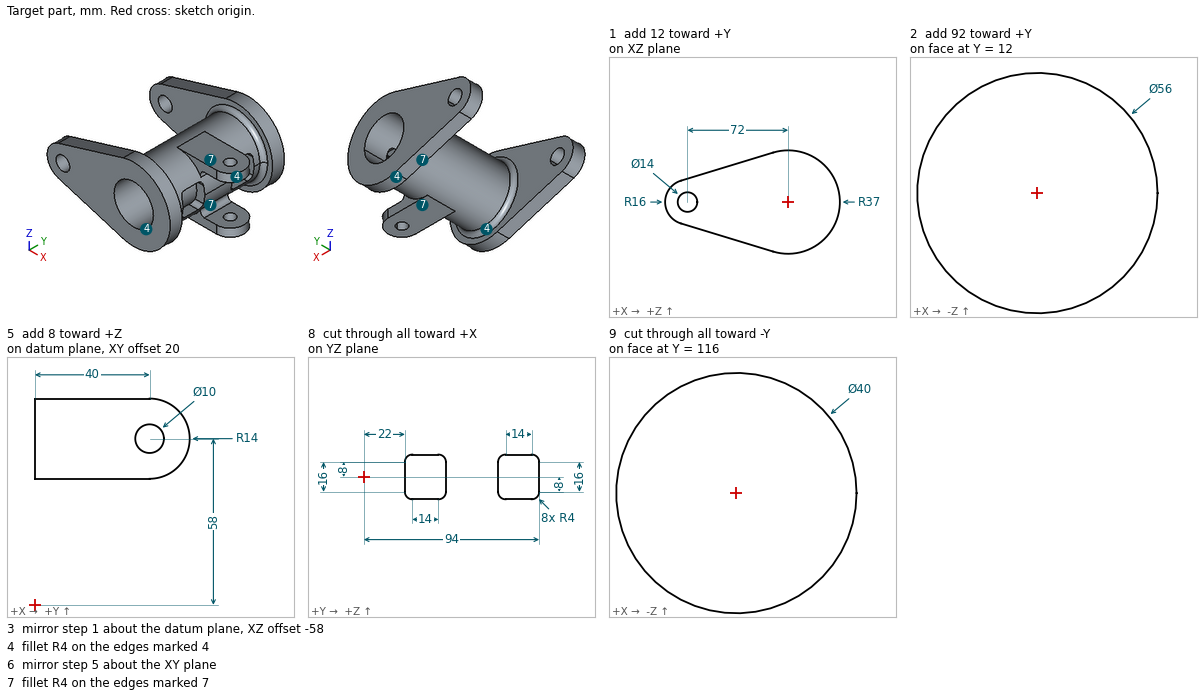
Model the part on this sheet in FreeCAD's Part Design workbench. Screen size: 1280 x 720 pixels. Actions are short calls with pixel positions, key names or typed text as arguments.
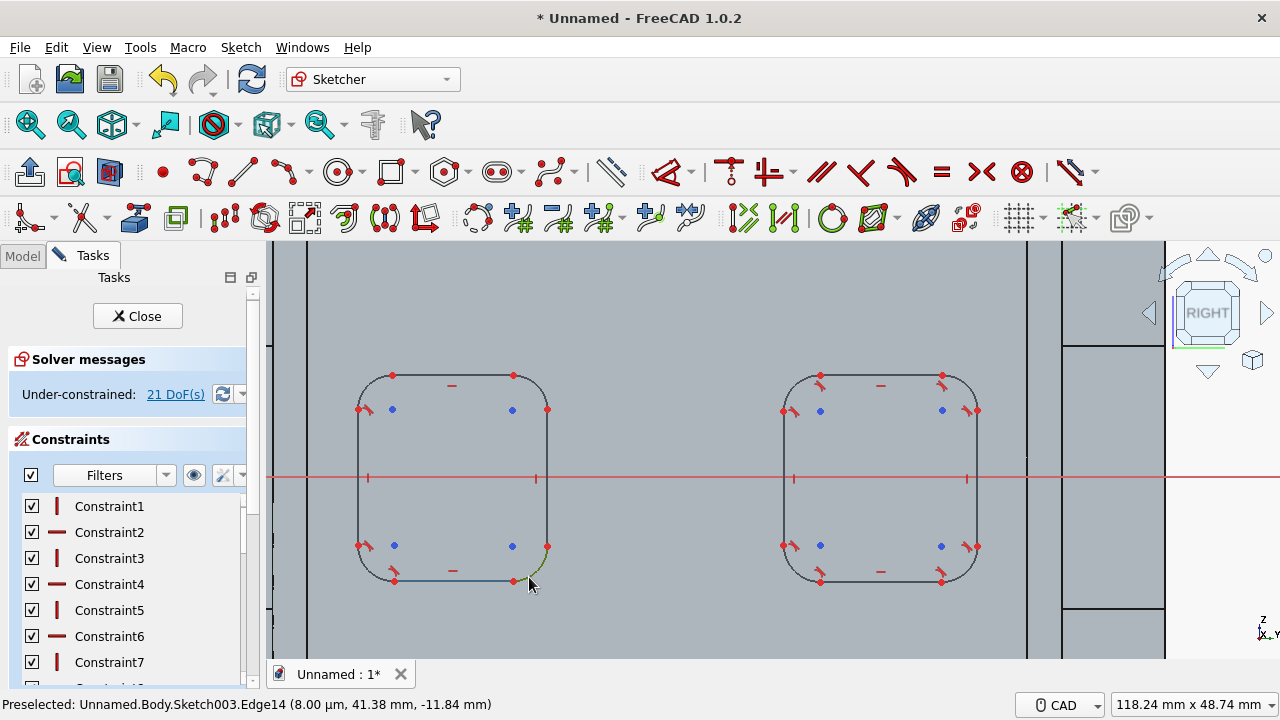
key(t)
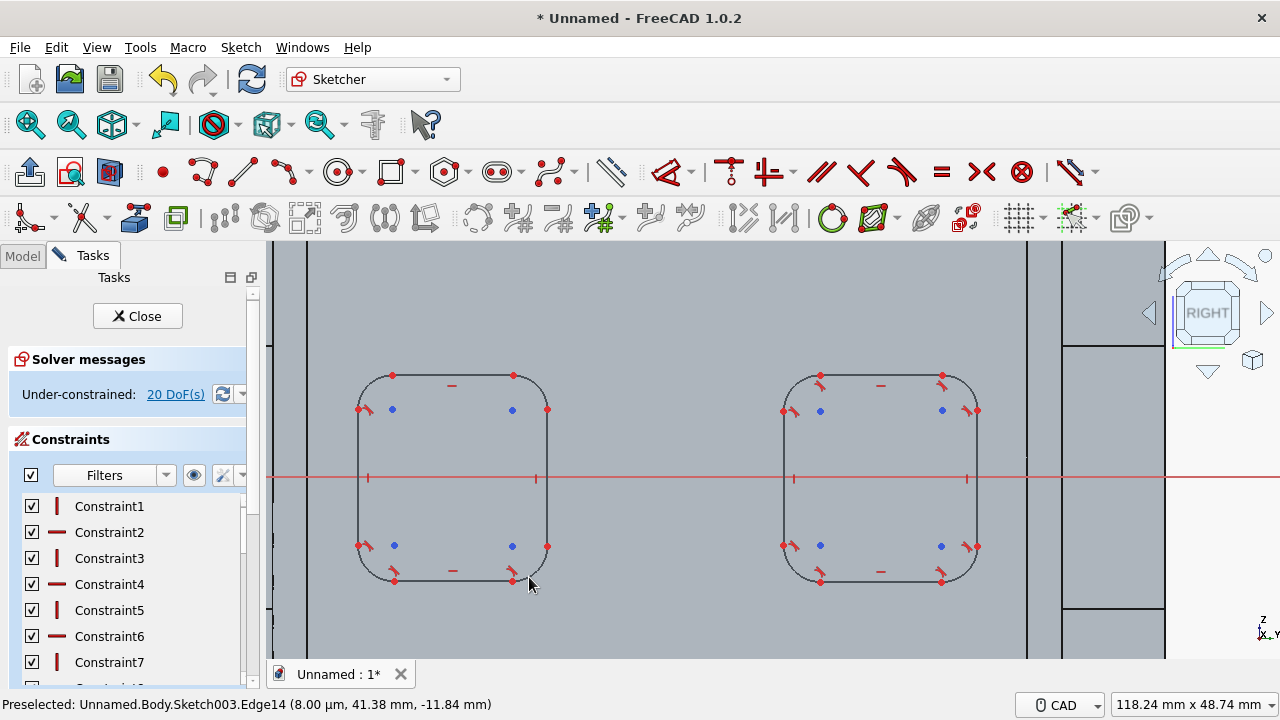
click(547, 506)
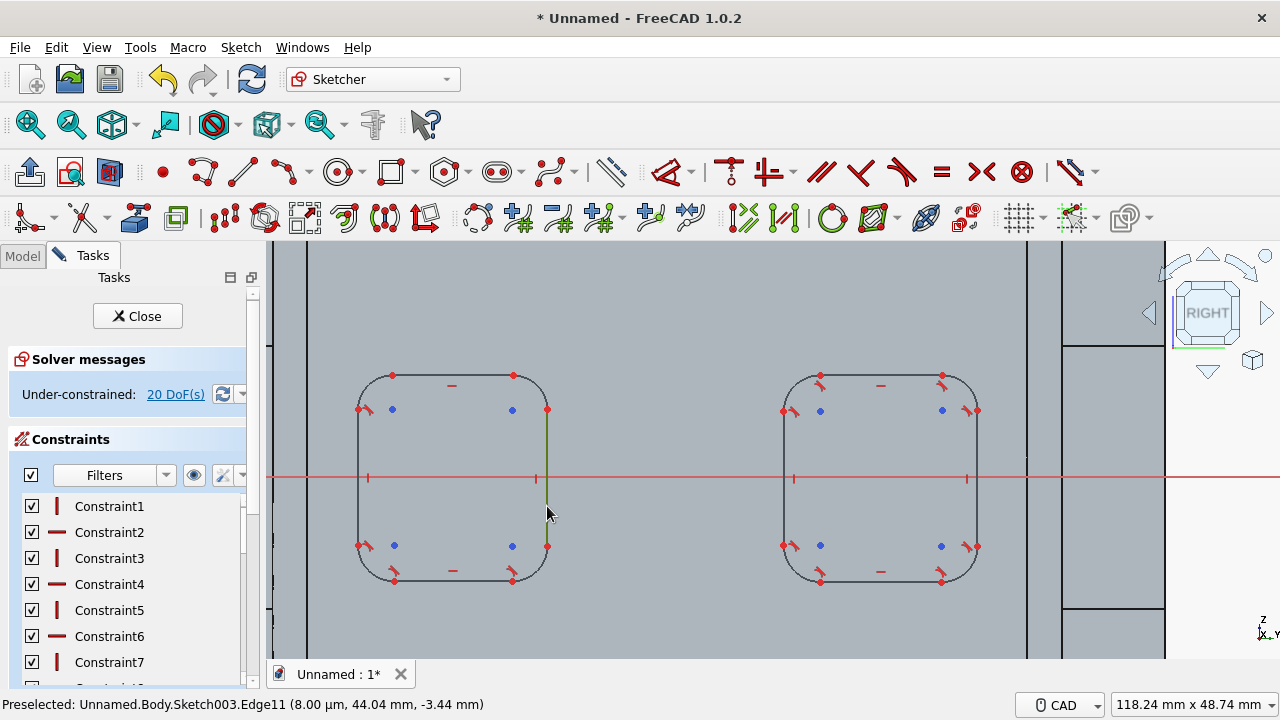
click(528, 578)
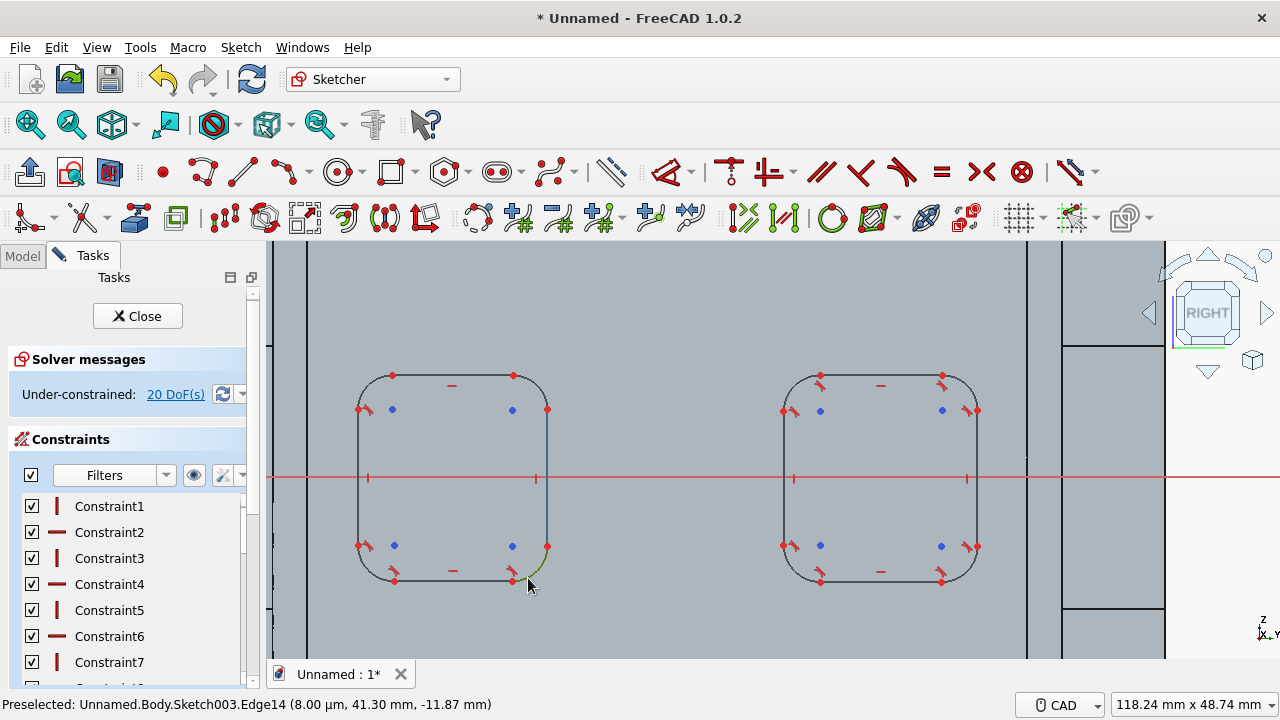
click(902, 172)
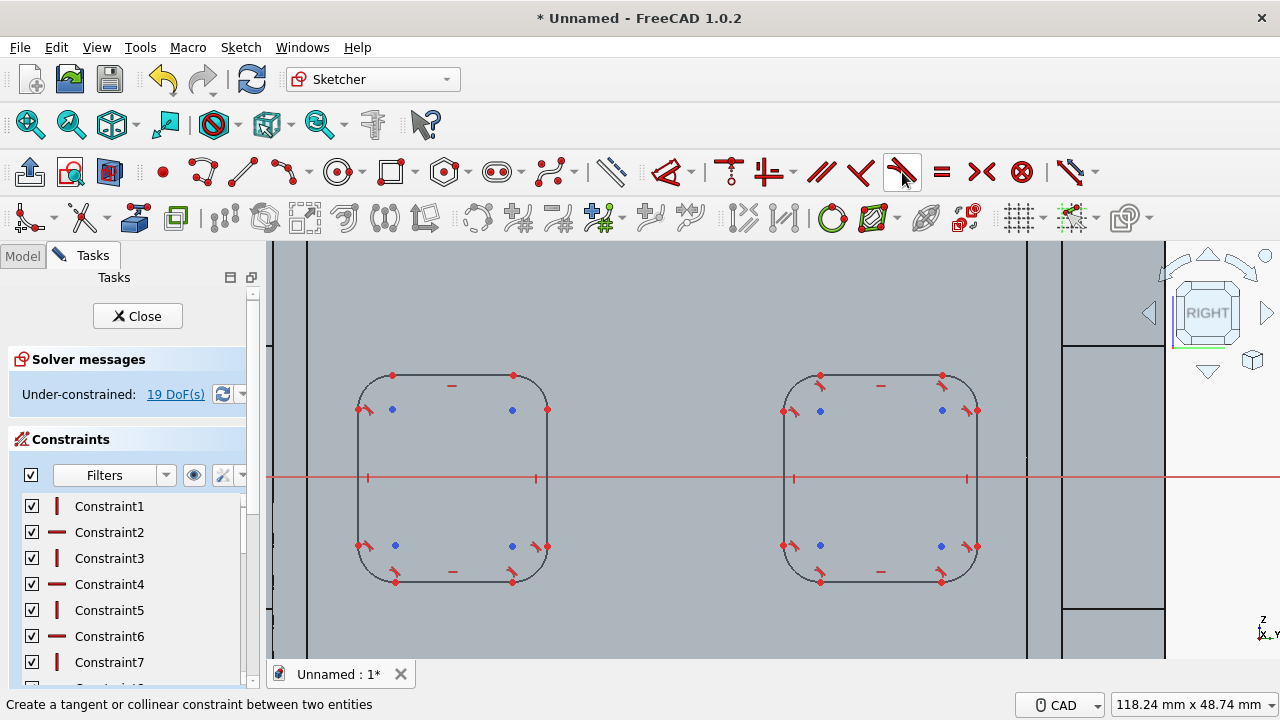
click(547, 506)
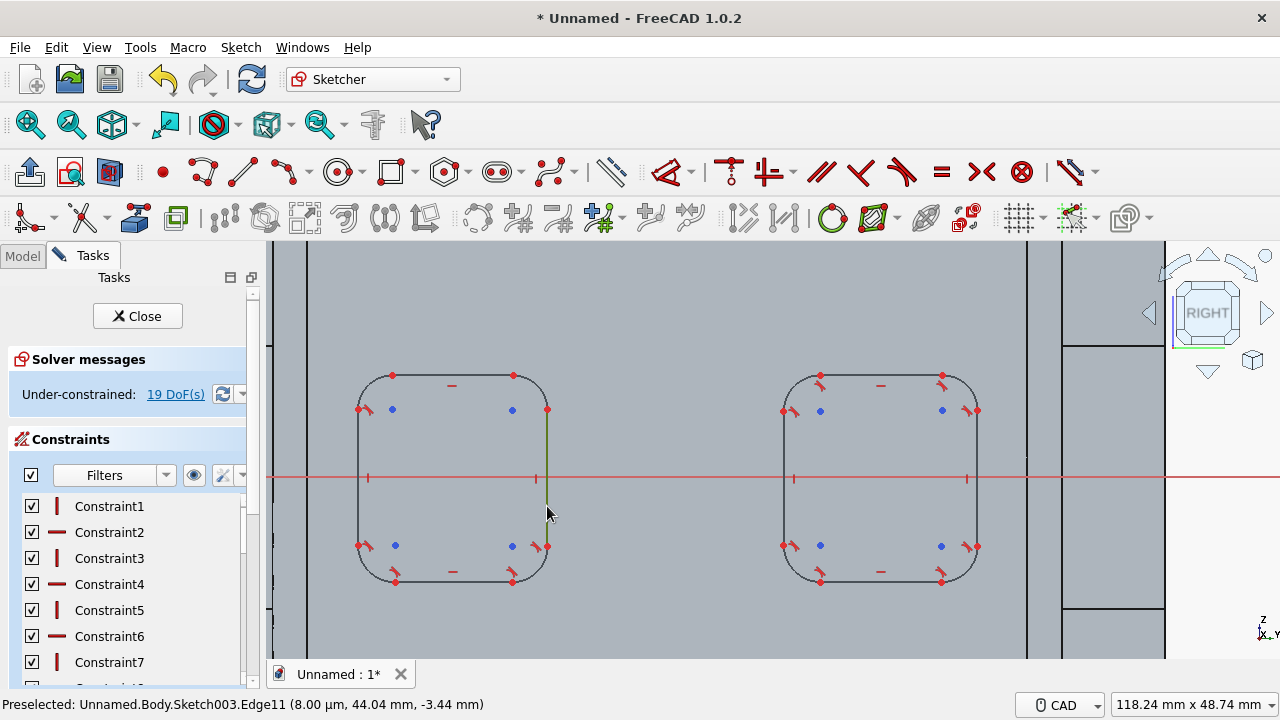
click(544, 394)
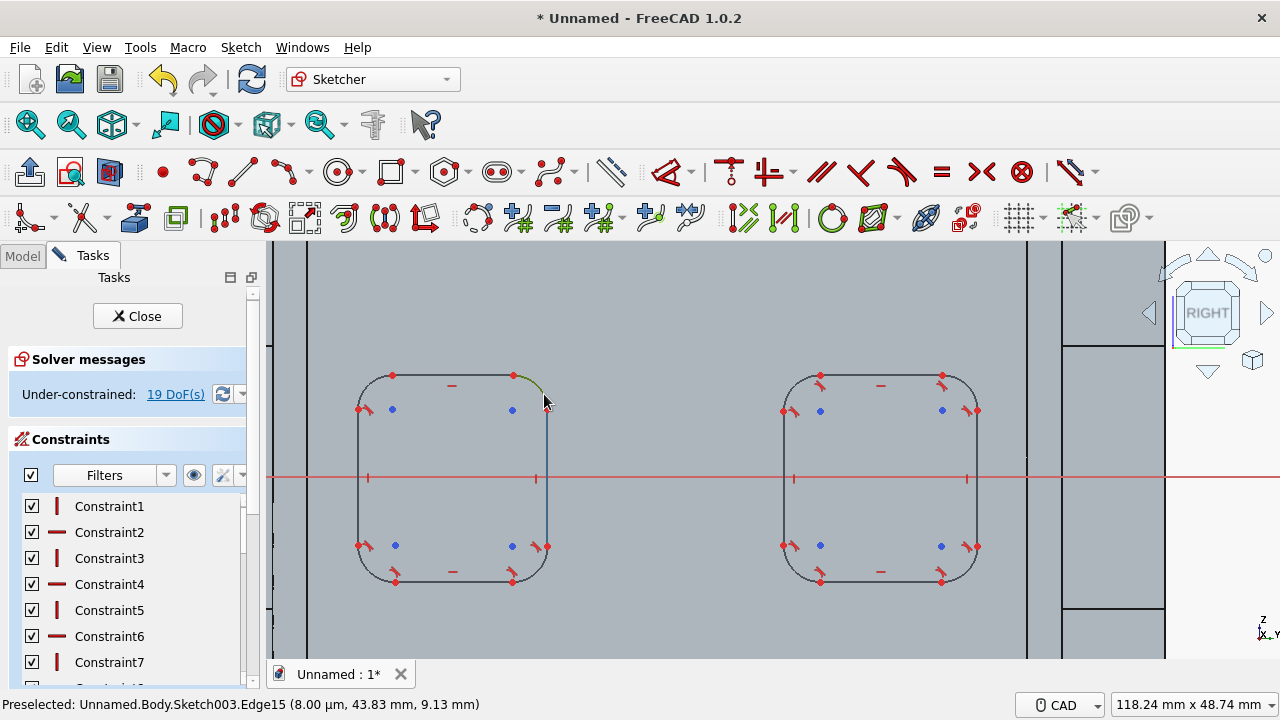
key(t)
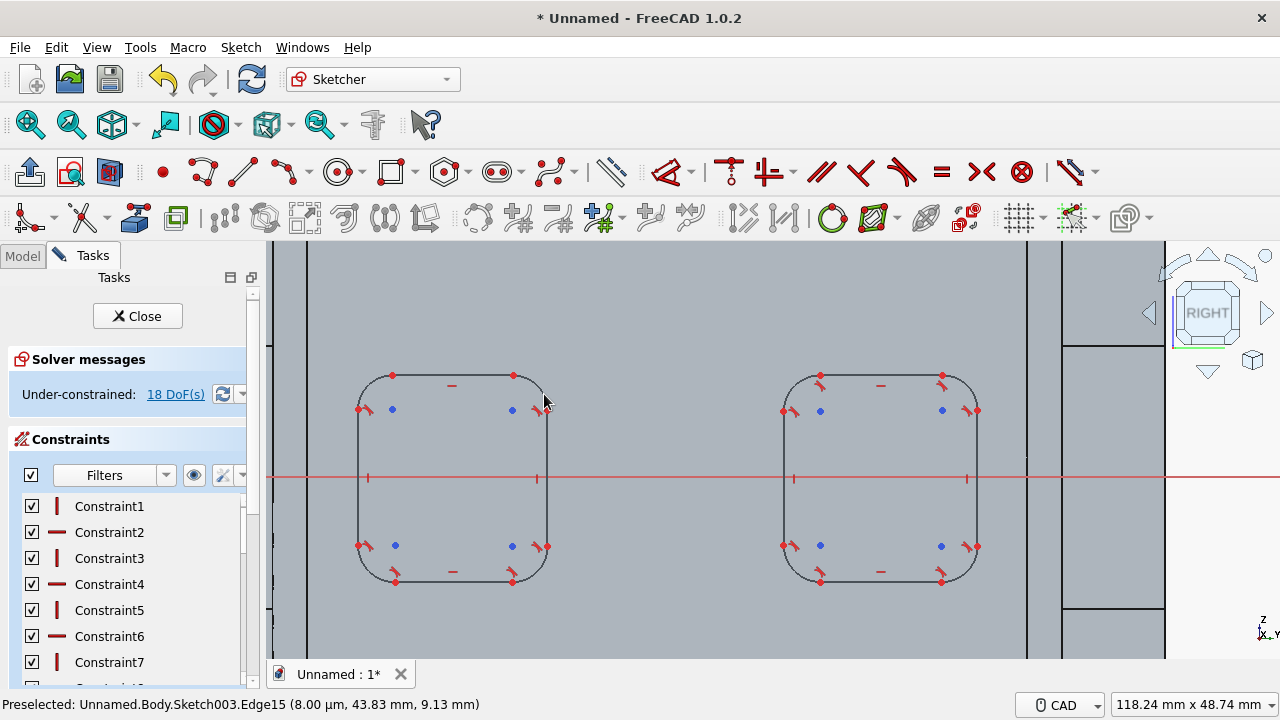
click(477, 375)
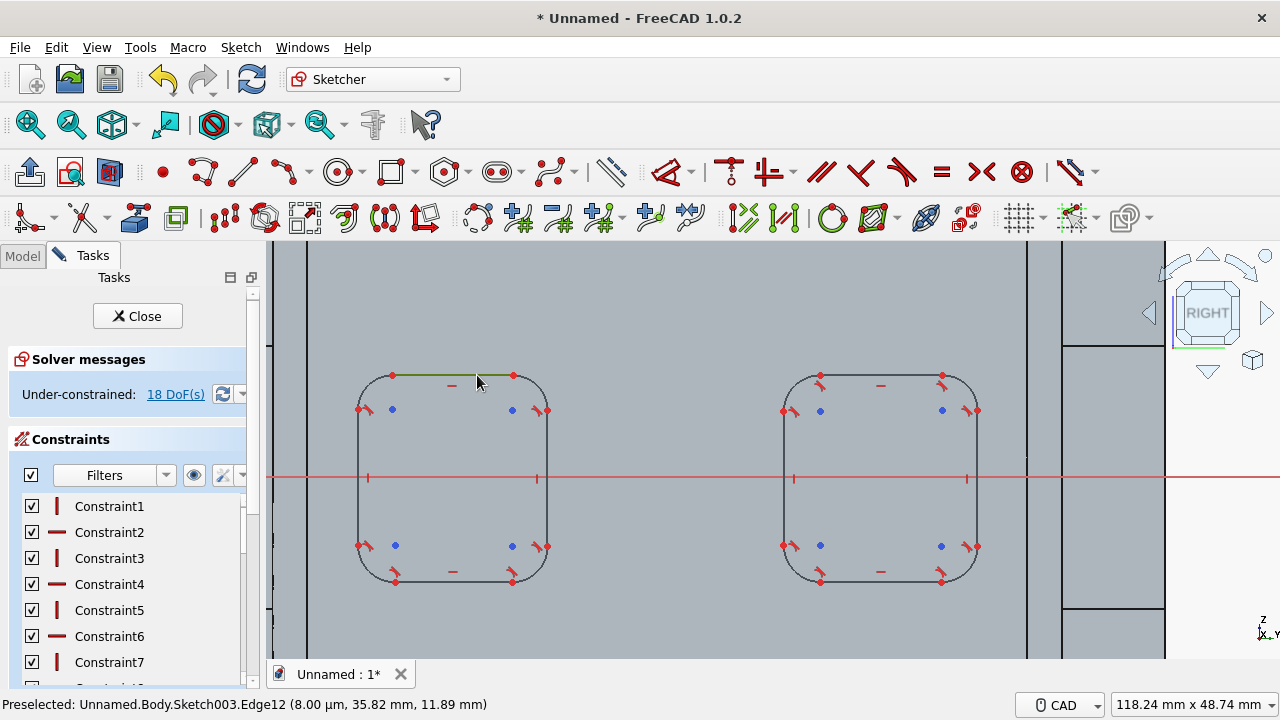
click(544, 395)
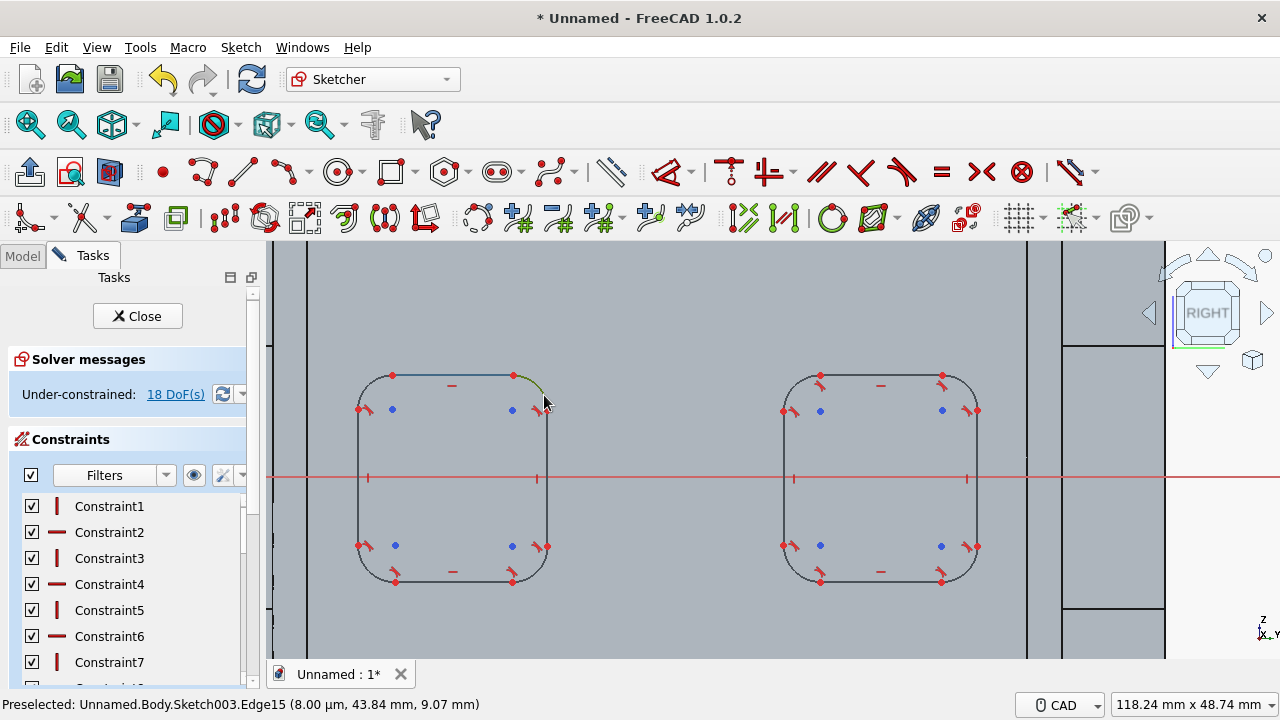
click(902, 172)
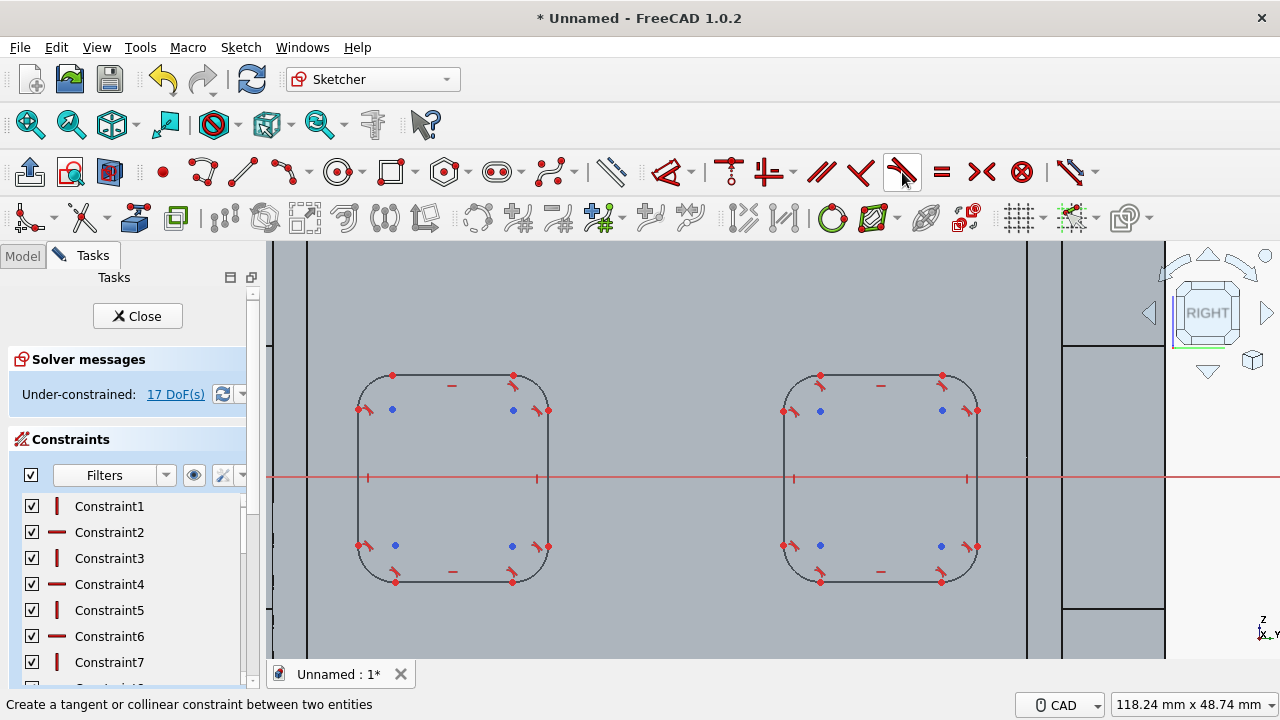
click(477, 375)